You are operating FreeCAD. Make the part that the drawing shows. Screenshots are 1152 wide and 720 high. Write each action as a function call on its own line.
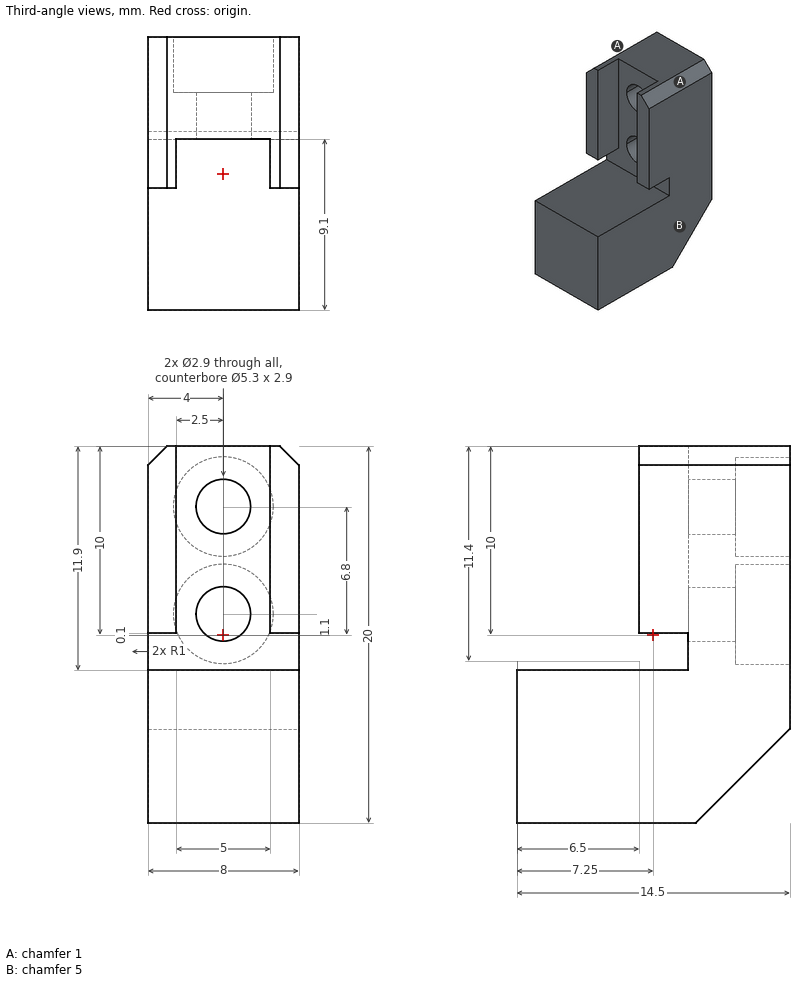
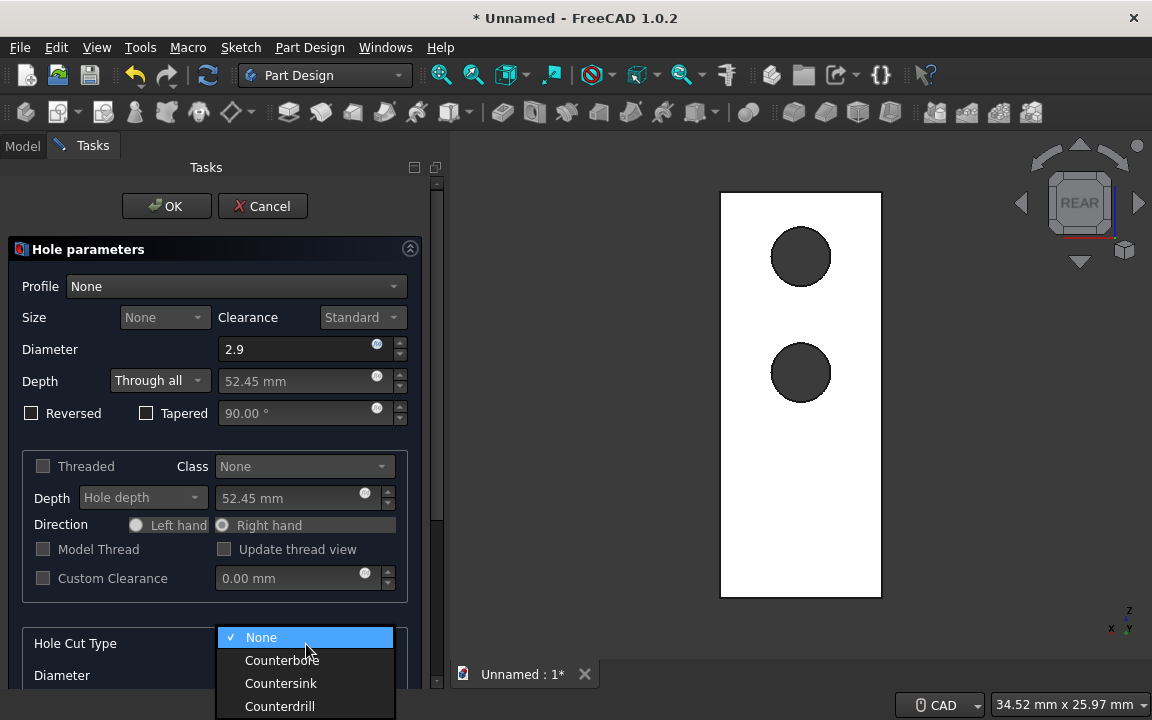
click(304, 660)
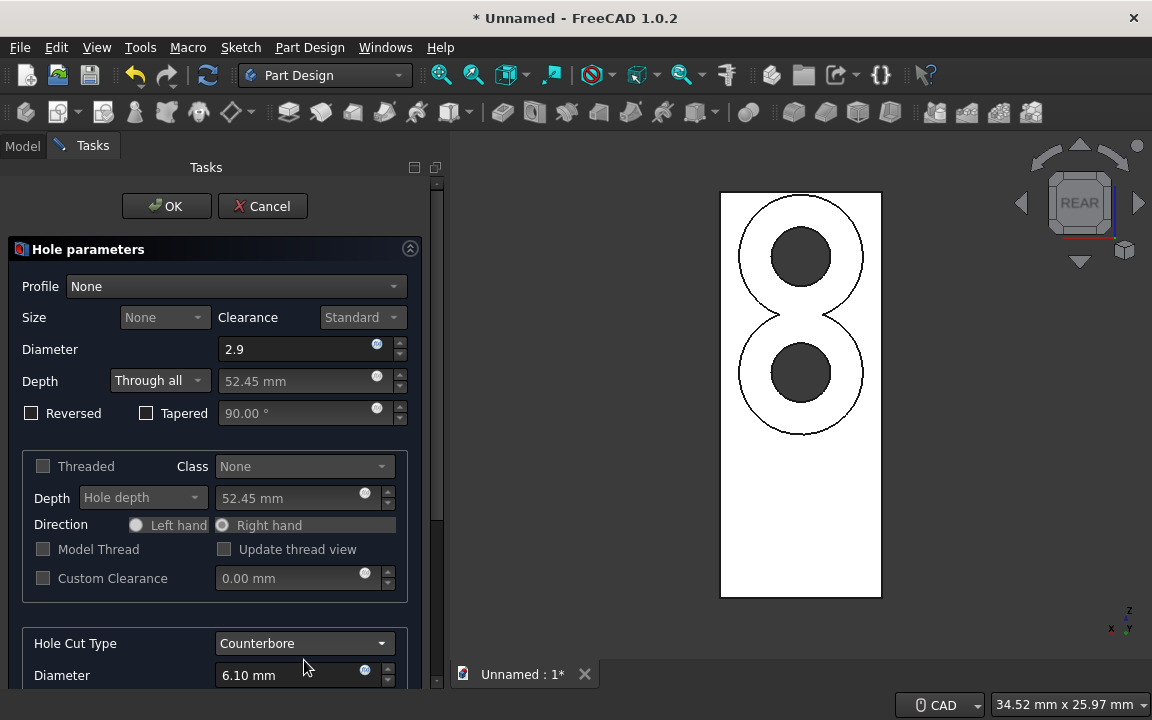
triple_click(298, 675)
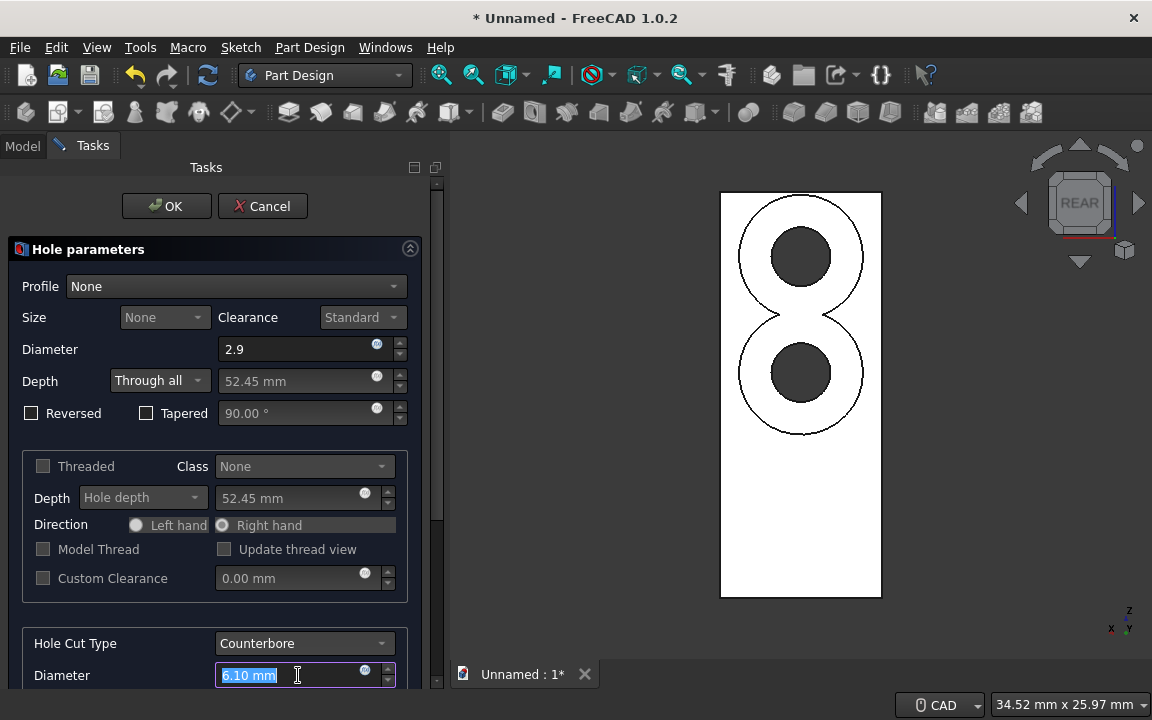
text(5.3)
key(Tab)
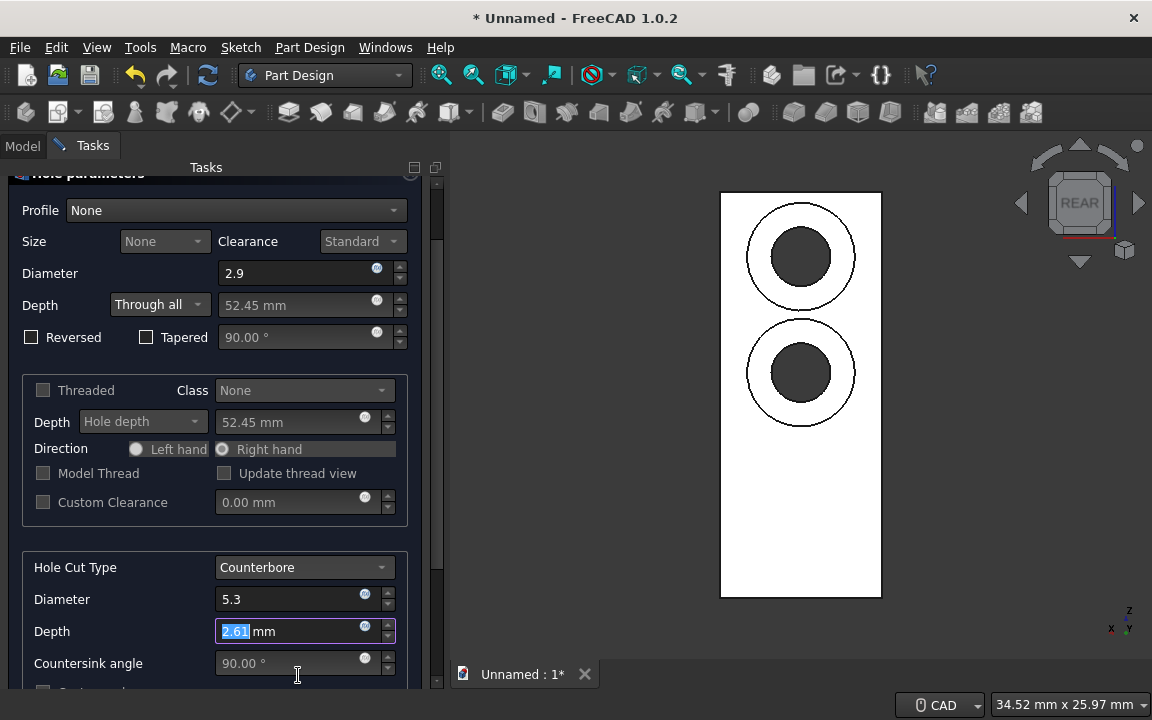
text(2.9)
key(Tab)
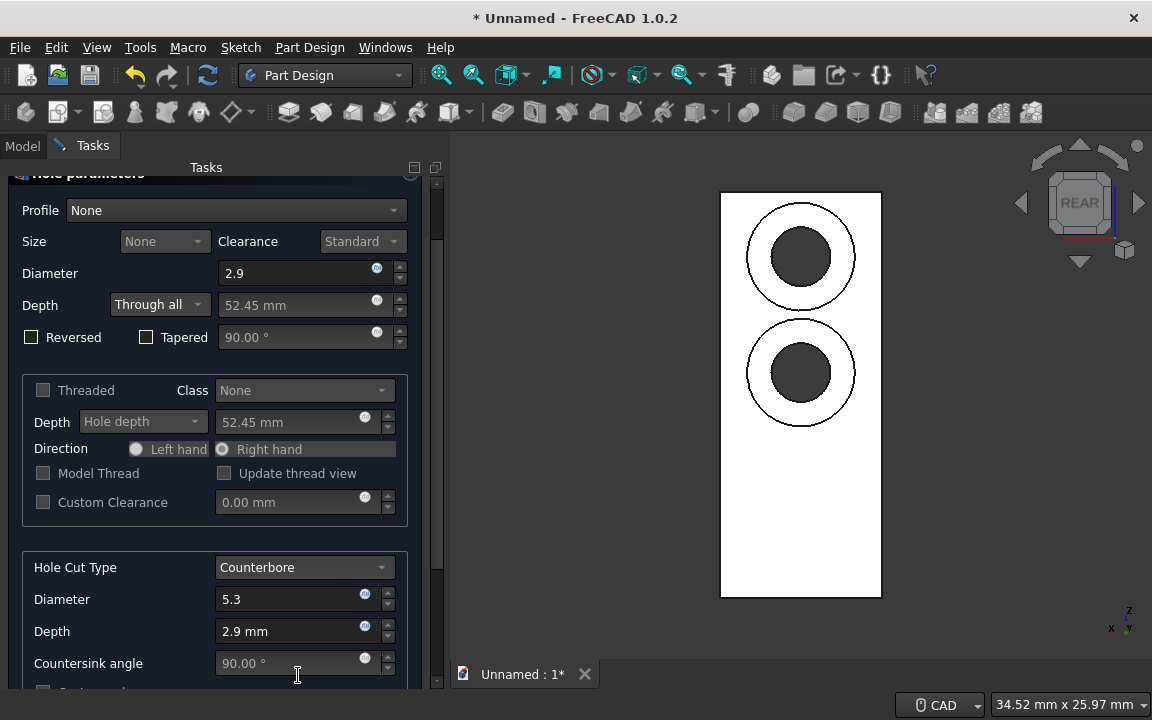
scroll(437, 432, up, 3)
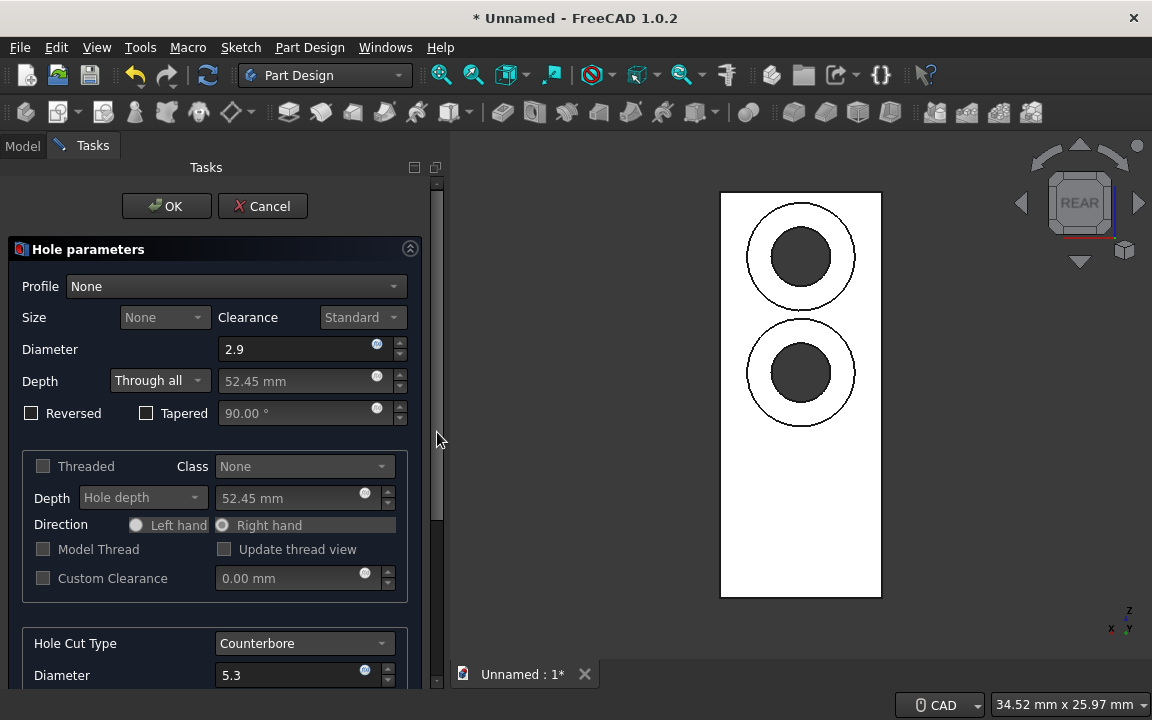
click(167, 206)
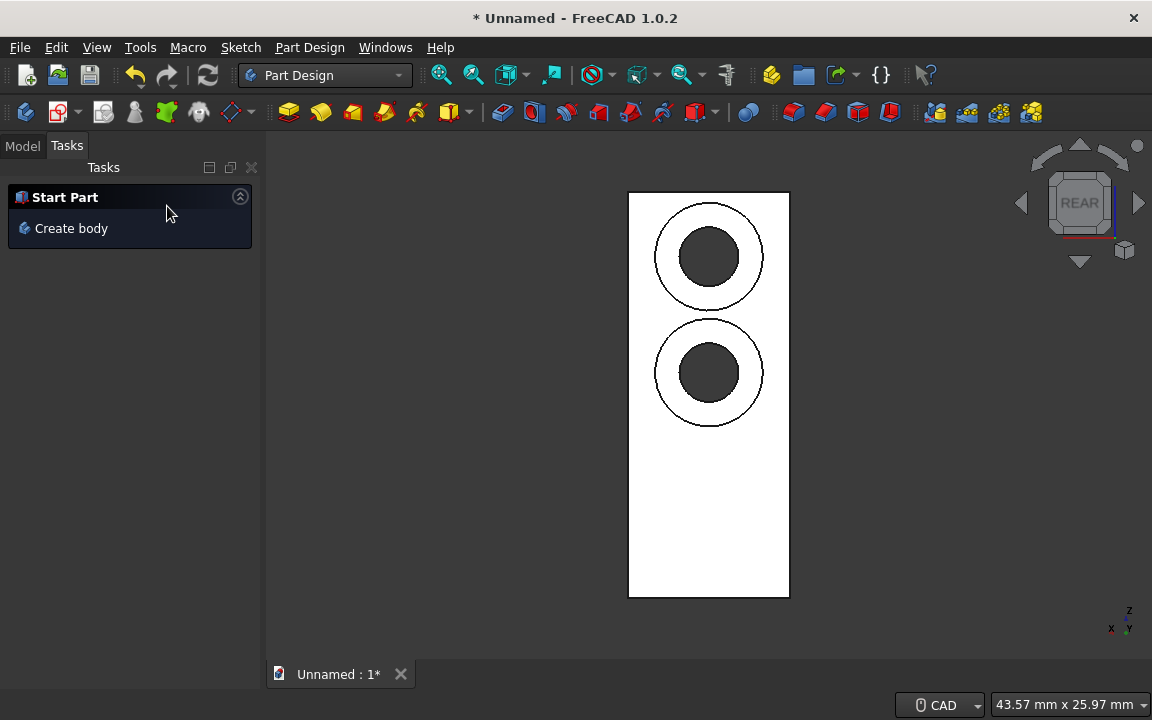
key(0)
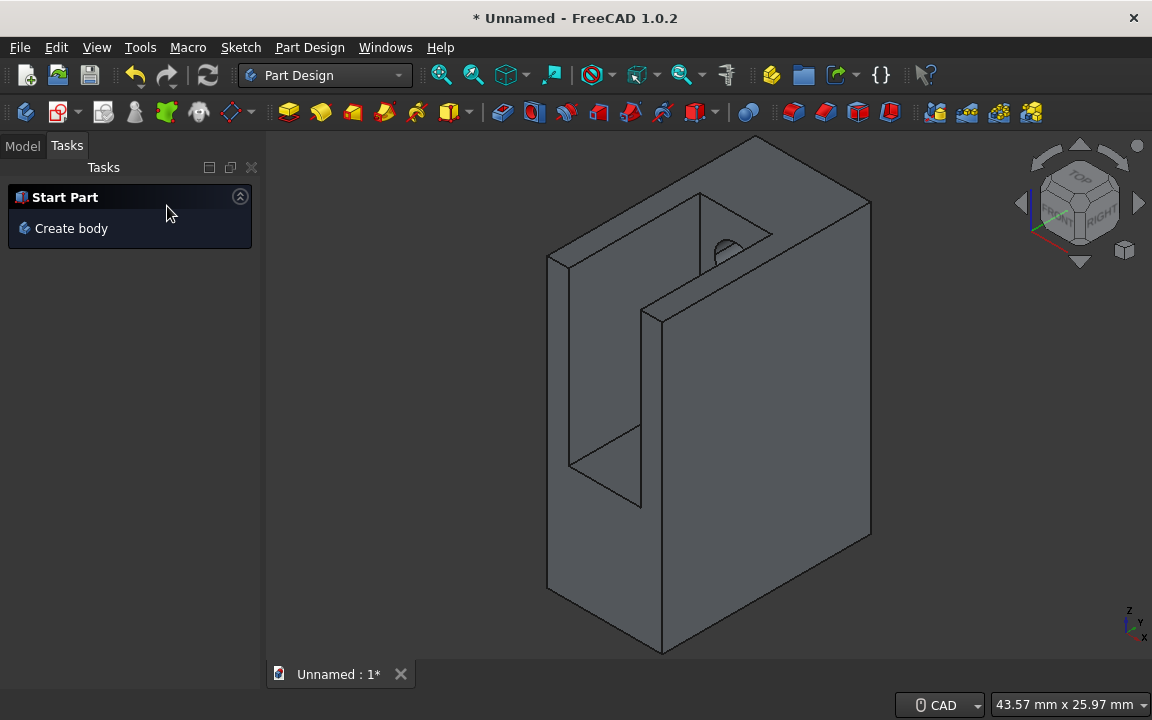
click(767, 427)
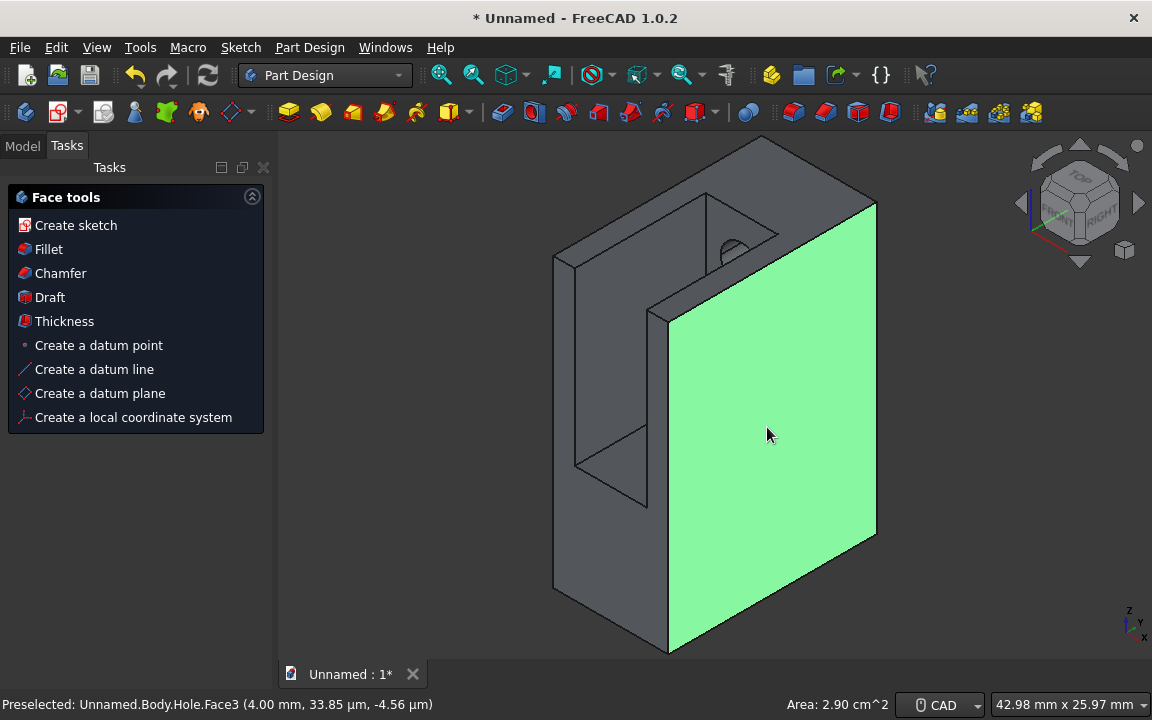
click(58, 112)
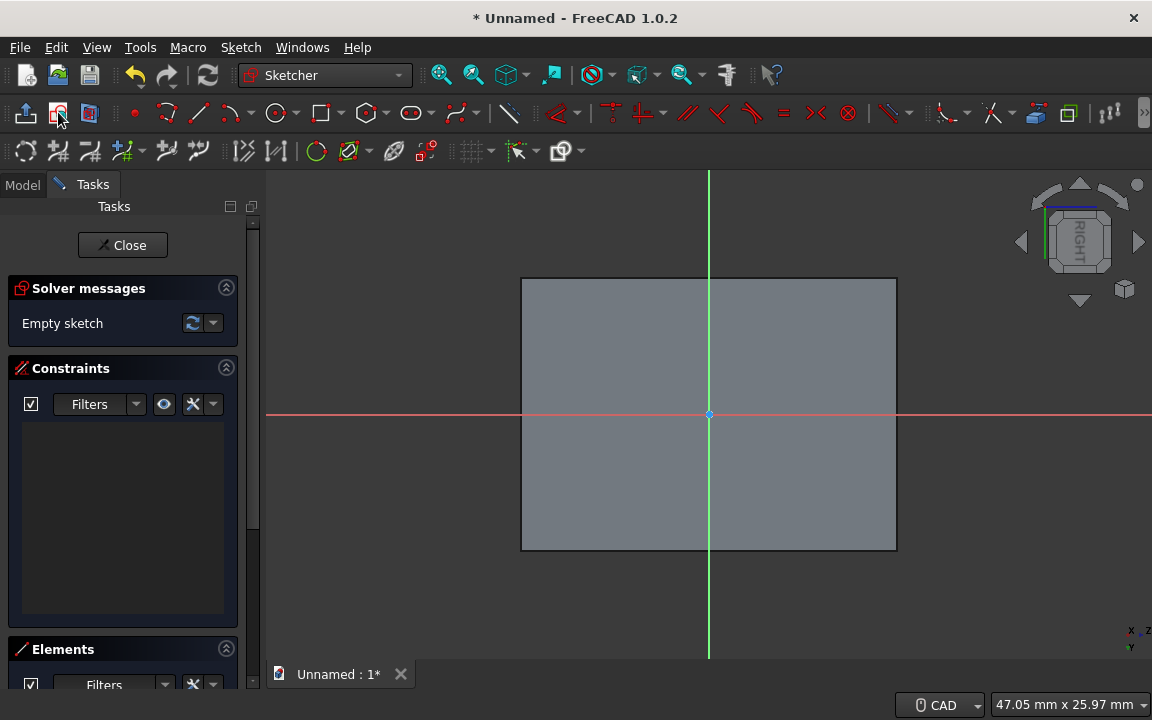
scroll(912, 291, up, 4)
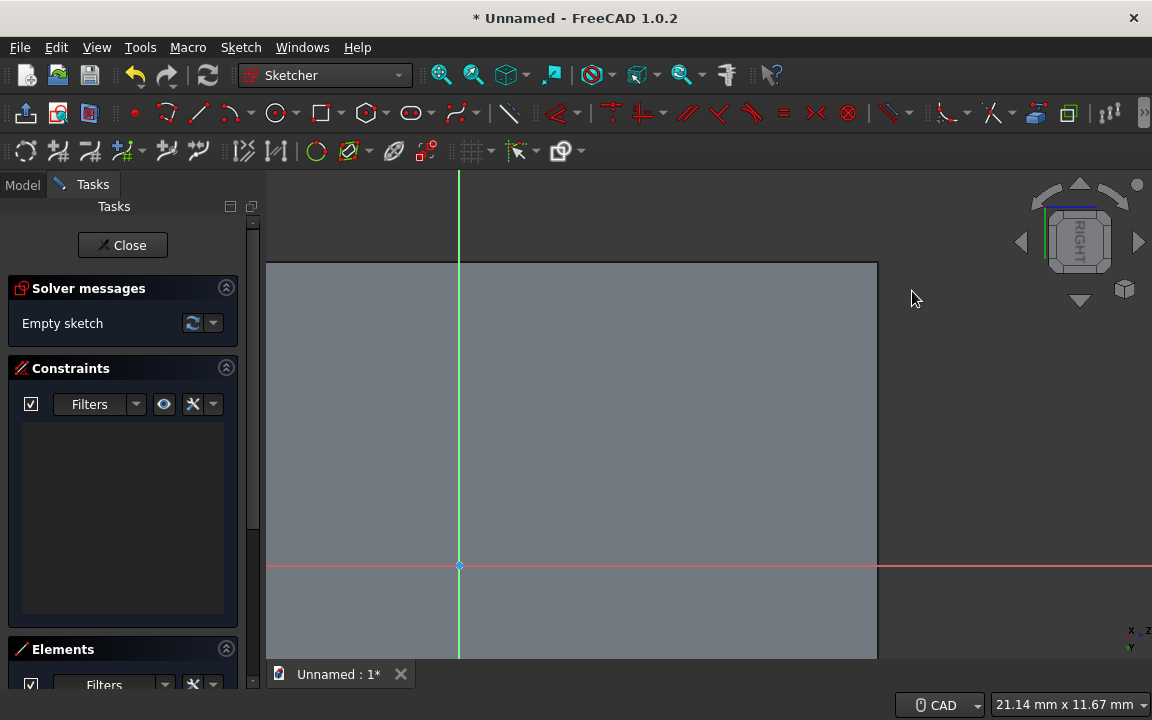
key(g)
key(r)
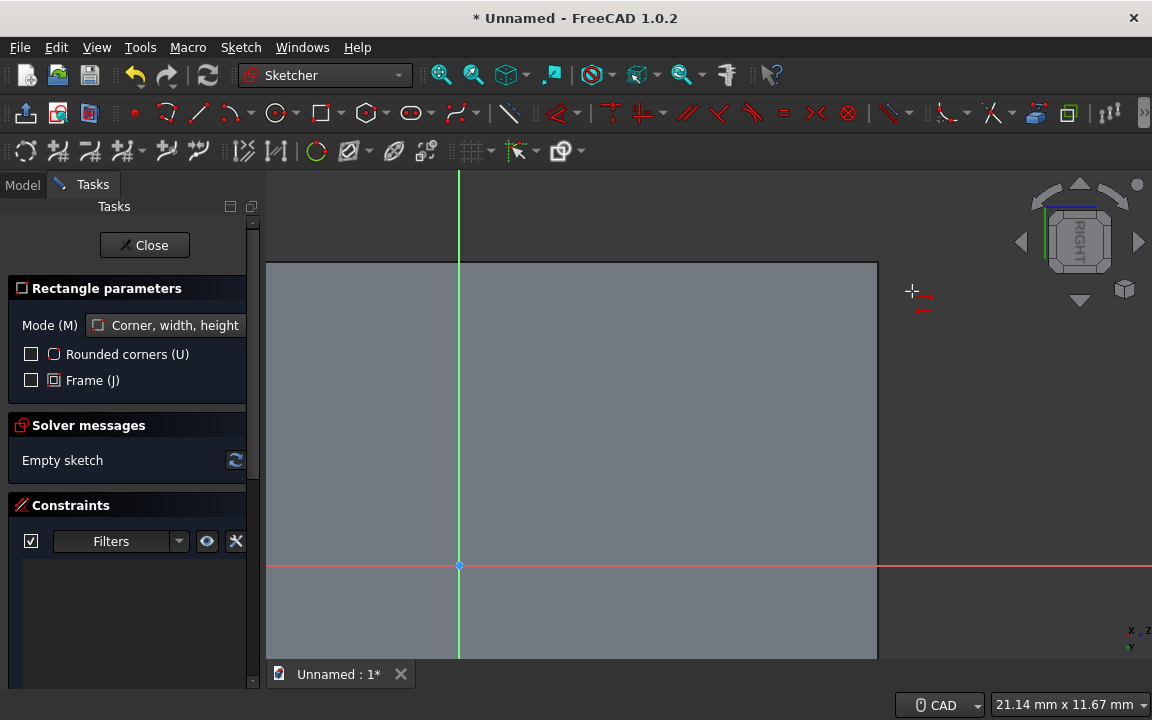
click(401, 262)
click(878, 534)
key(Escape)